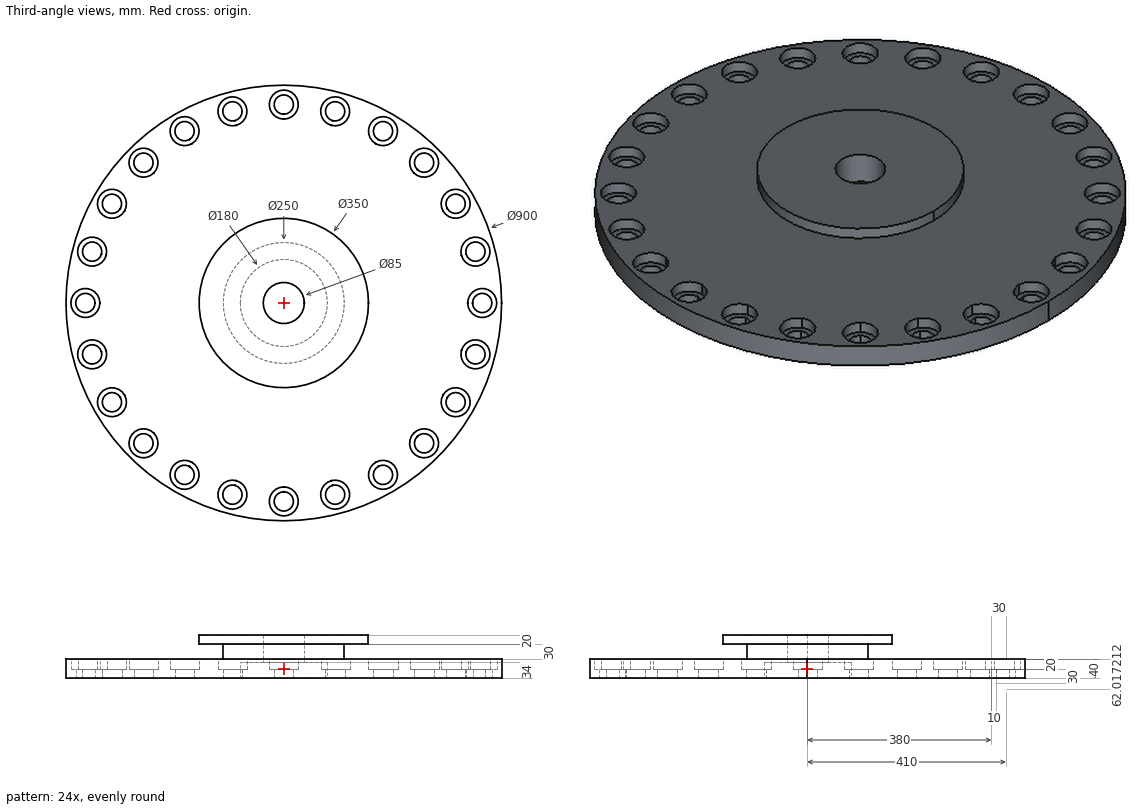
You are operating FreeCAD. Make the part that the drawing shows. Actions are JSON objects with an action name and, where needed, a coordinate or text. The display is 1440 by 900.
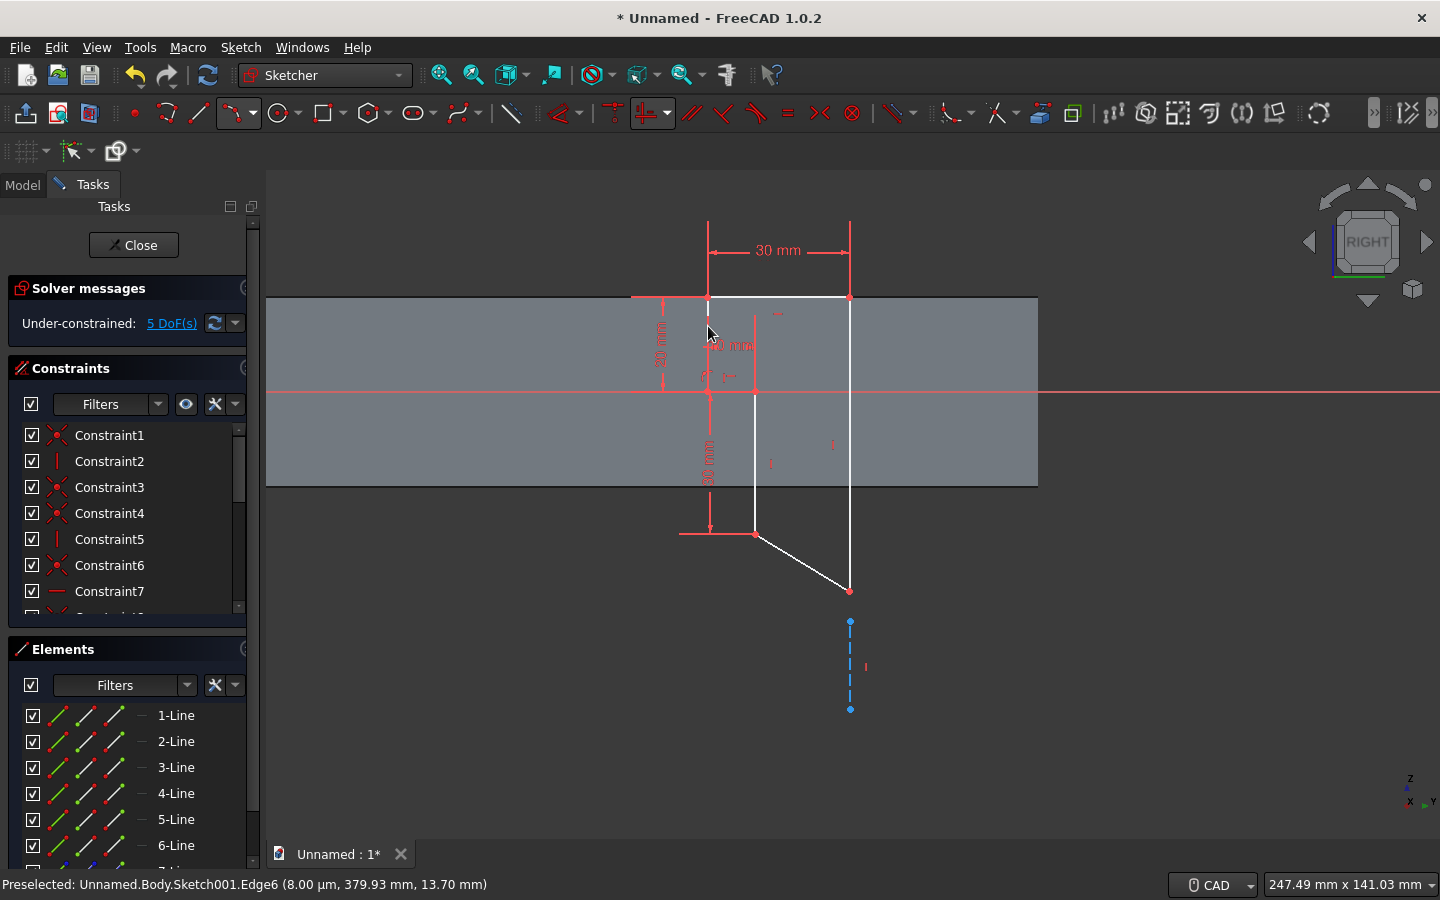
{"action": "left_click", "coordinate": [708, 392]}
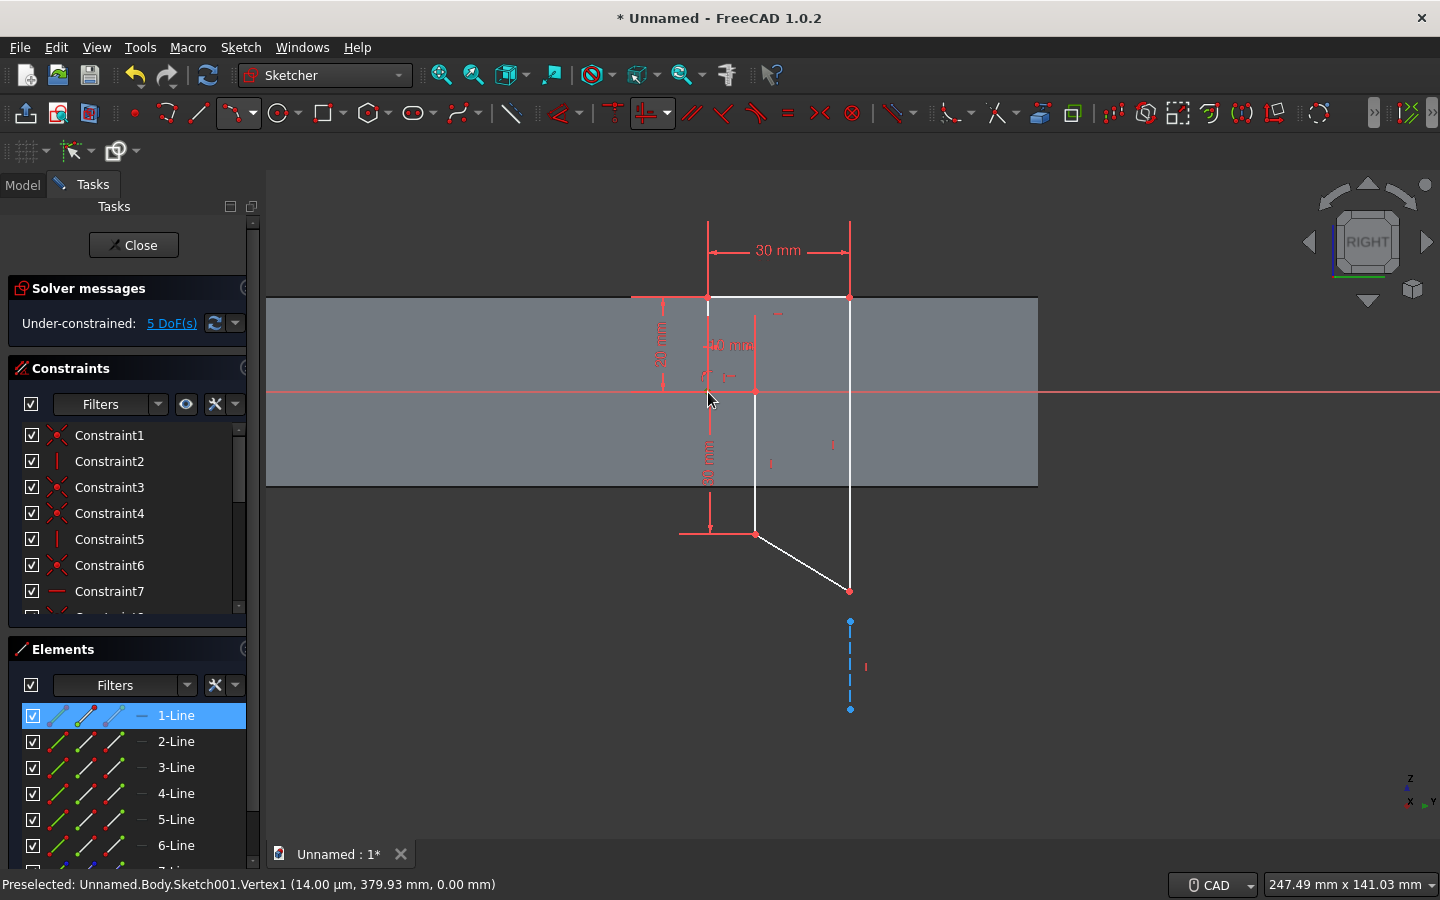
{"action": "left_click", "coordinate": [582, 114]}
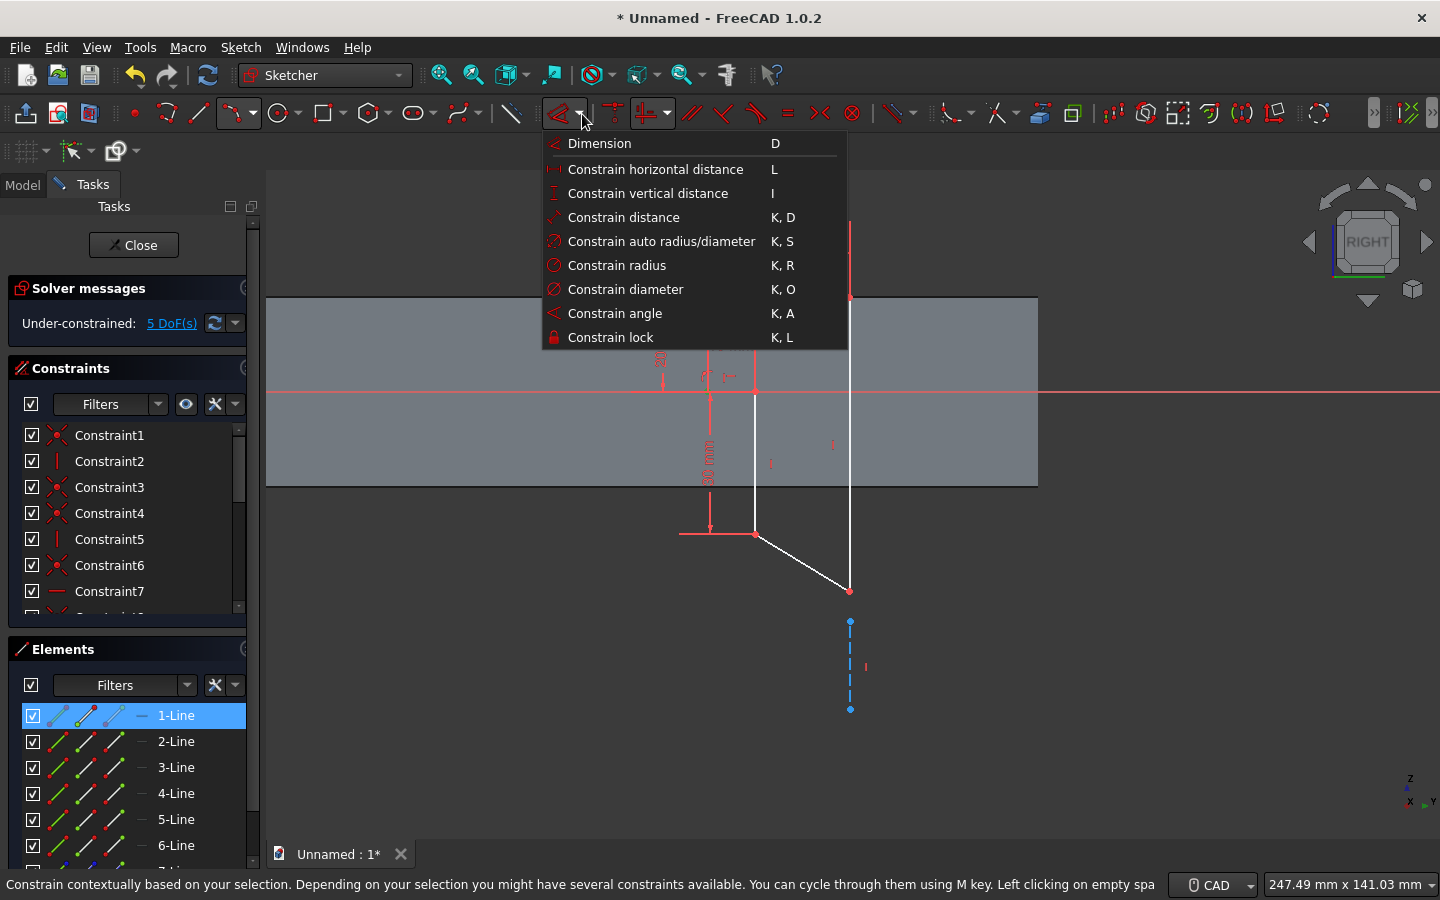
{"action": "left_click", "coordinate": [695, 169]}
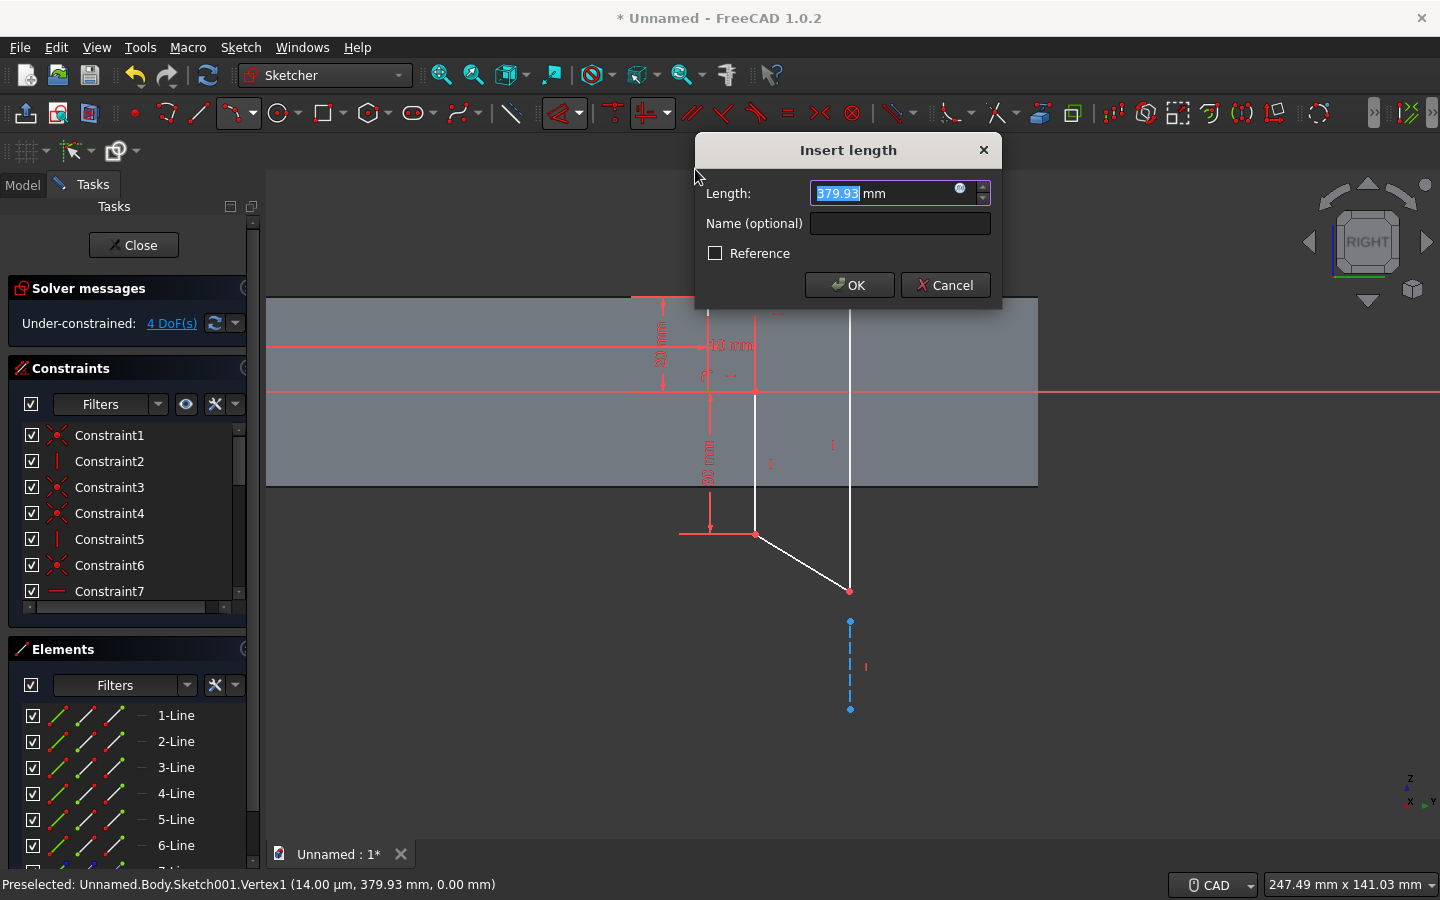
{"action": "type", "text": "380"}
{"action": "key", "text": "Return"}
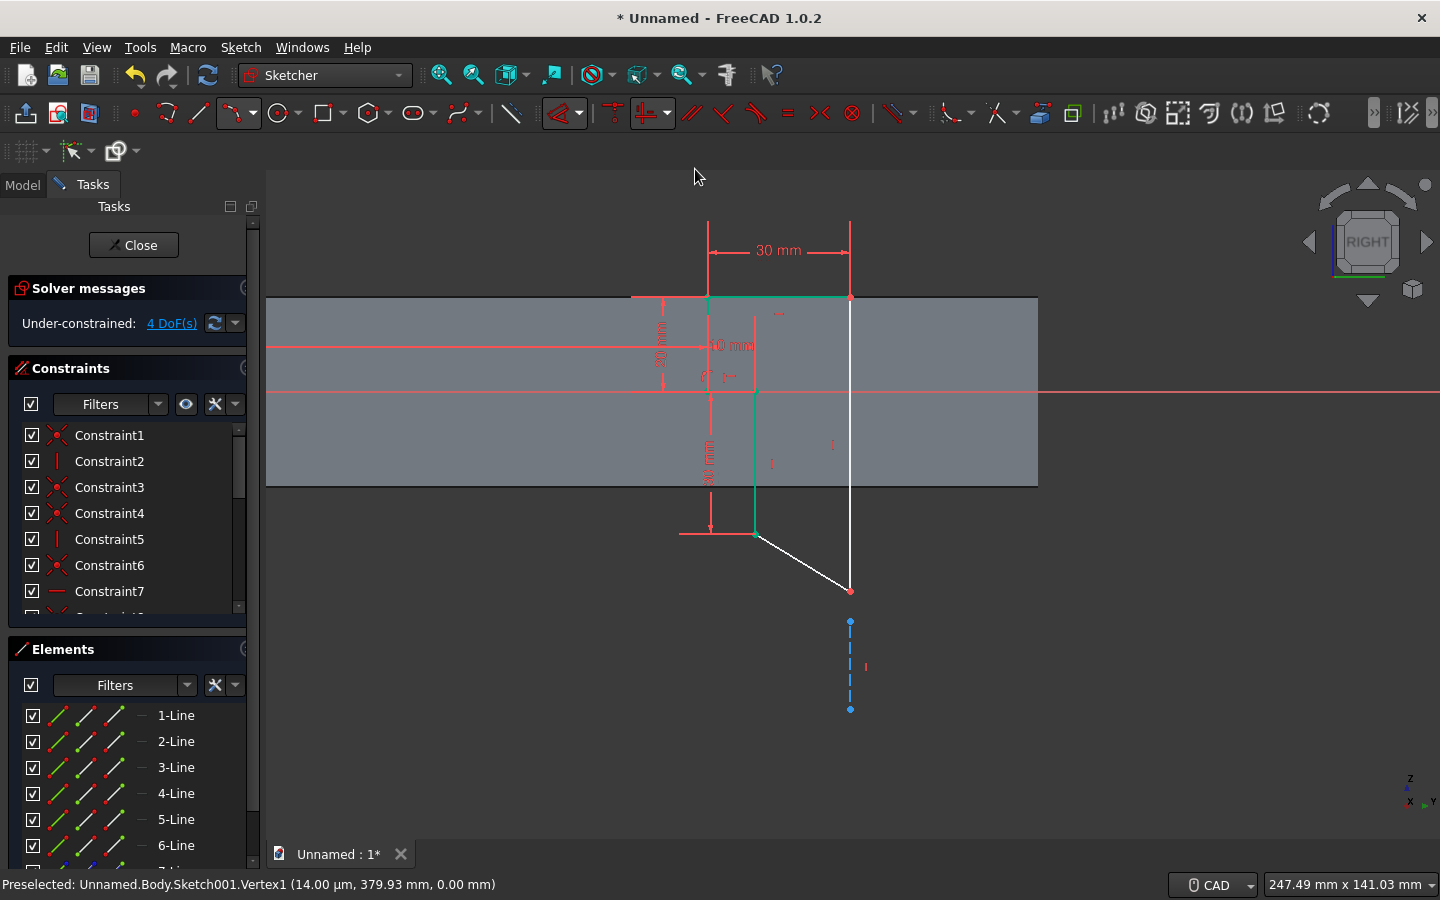
{"action": "left_click", "coordinate": [850, 622]}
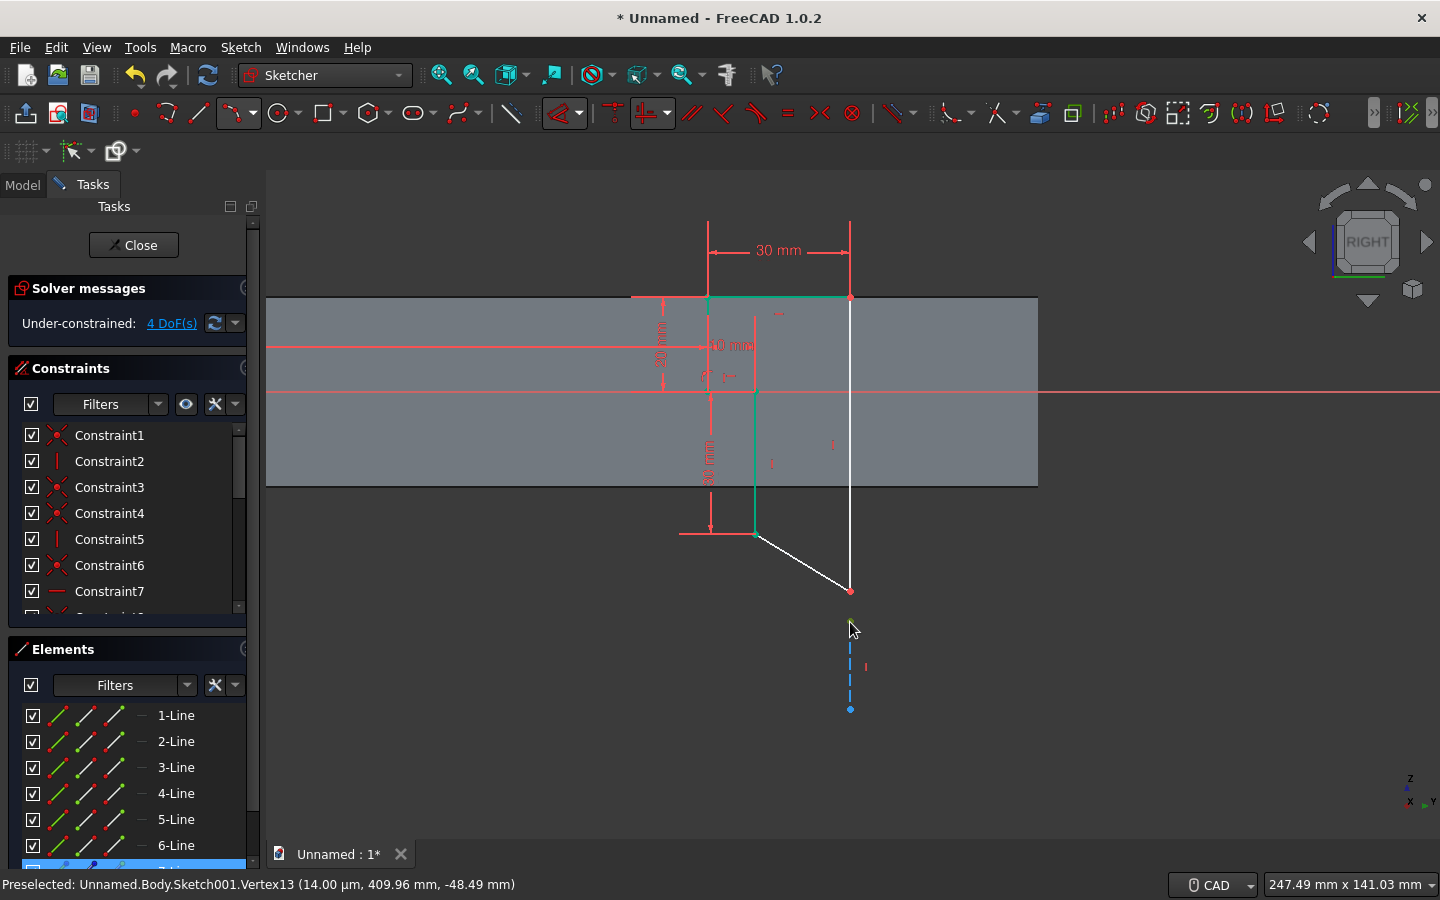
{"action": "left_click", "coordinate": [582, 114]}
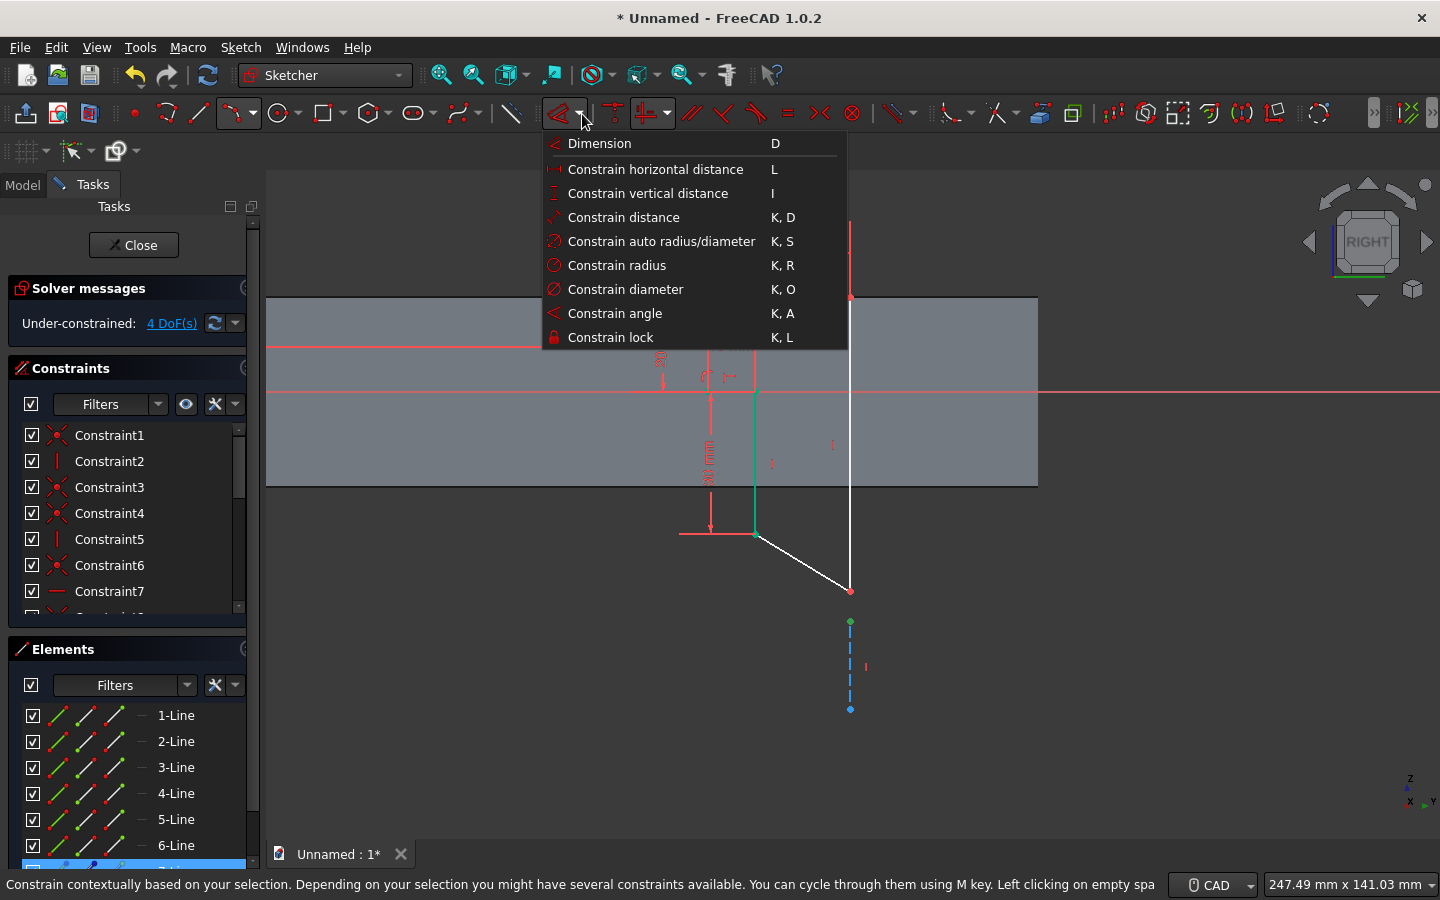
{"action": "left_click", "coordinate": [695, 169]}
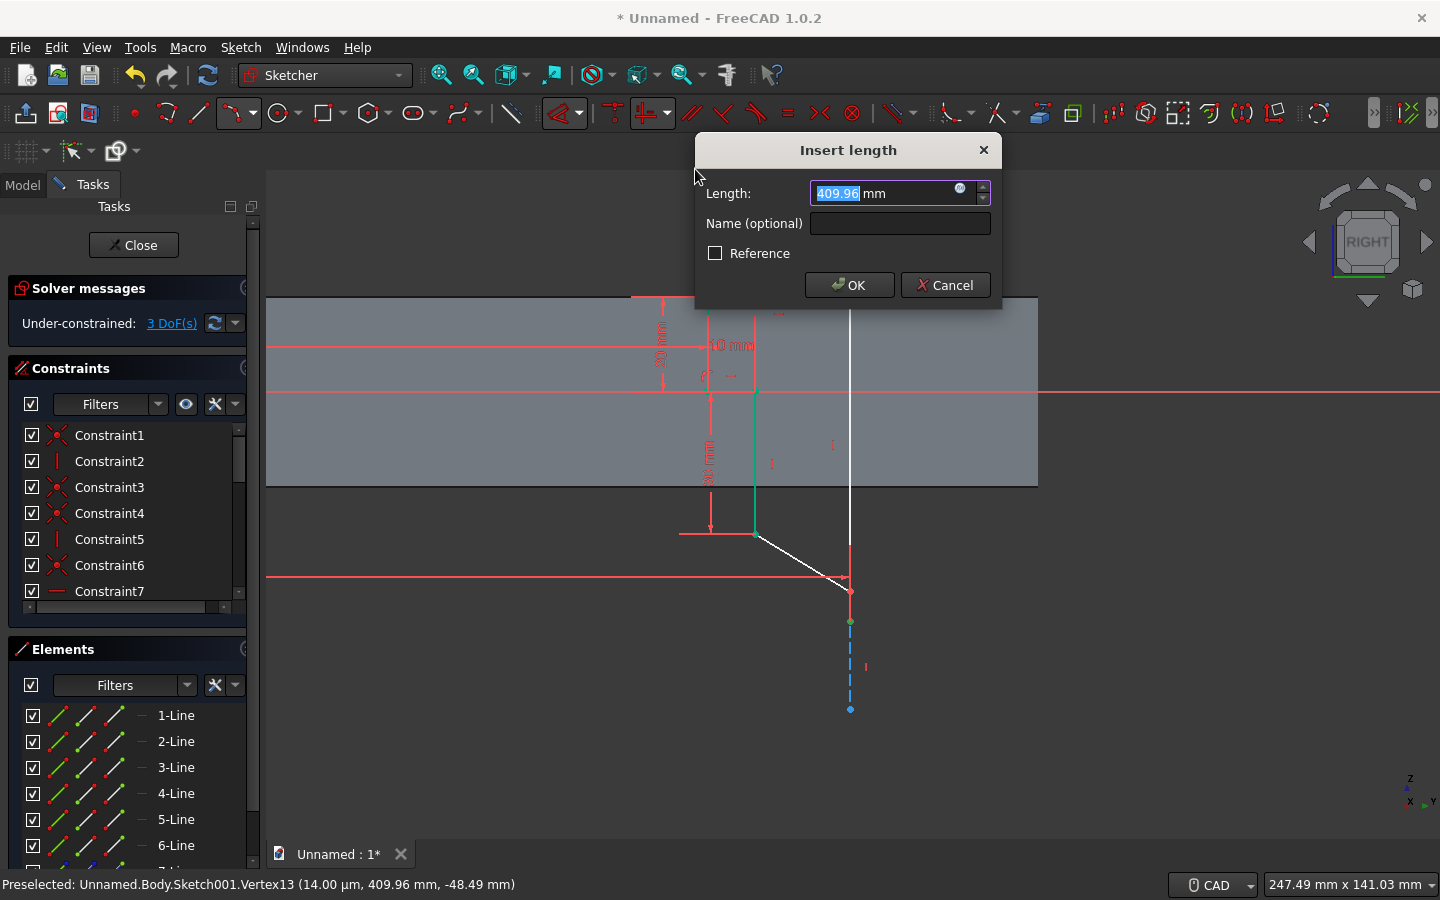
{"action": "type", "text": "410"}
{"action": "key", "text": "Return"}